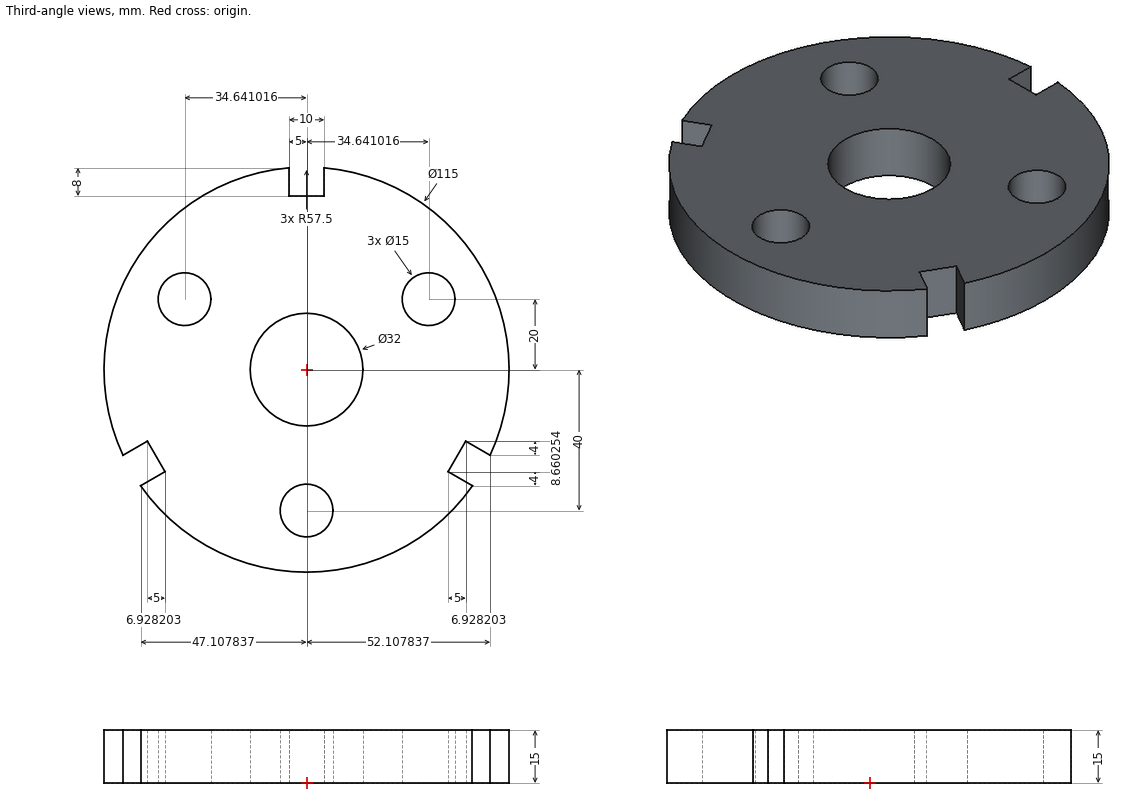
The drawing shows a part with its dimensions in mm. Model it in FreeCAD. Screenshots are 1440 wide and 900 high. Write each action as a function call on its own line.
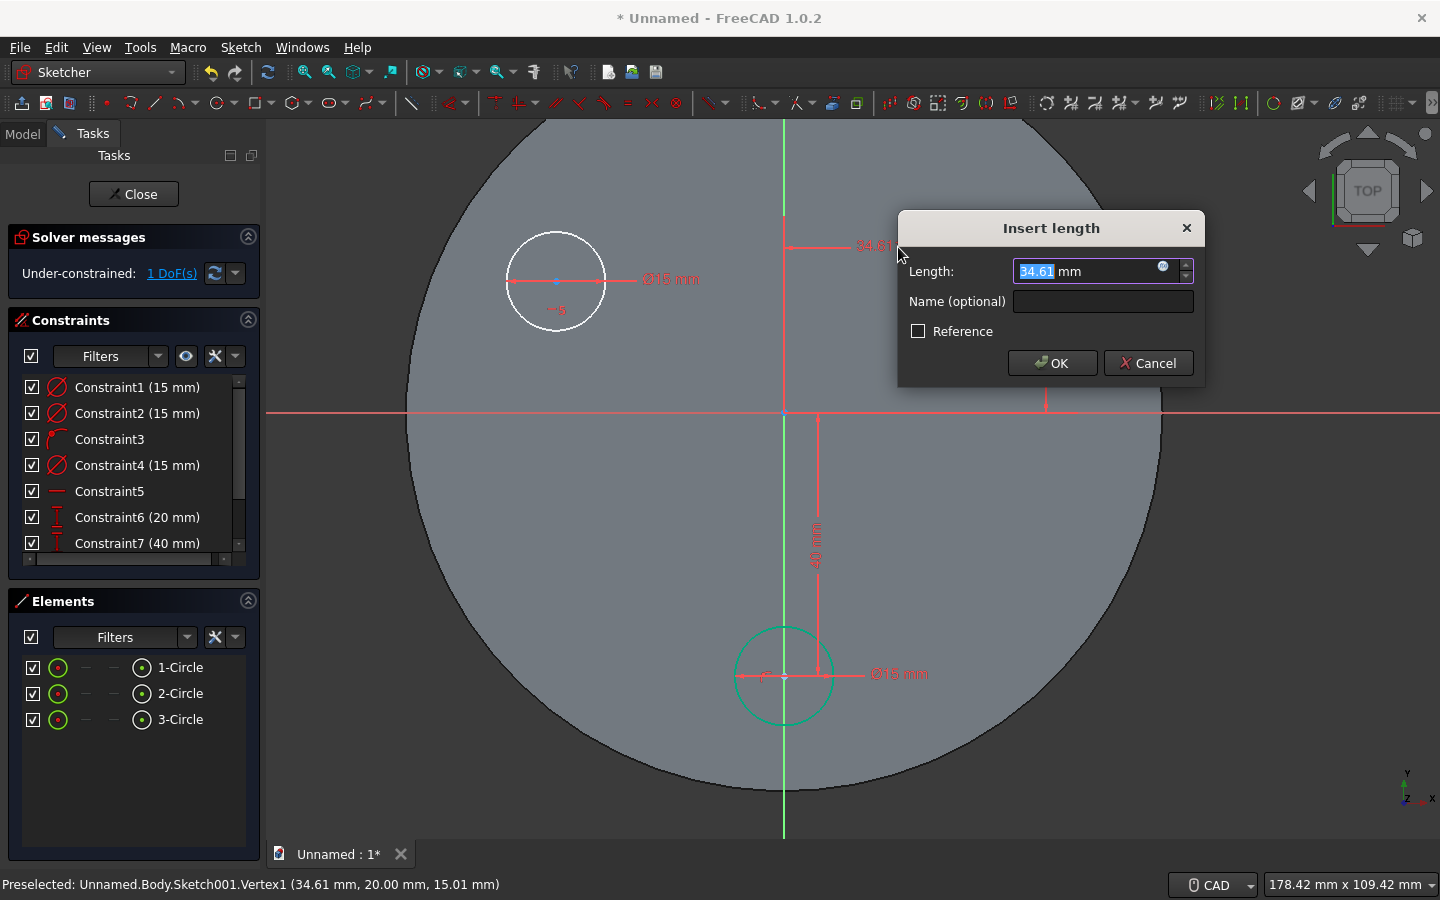
text(34.641016)
key(Return)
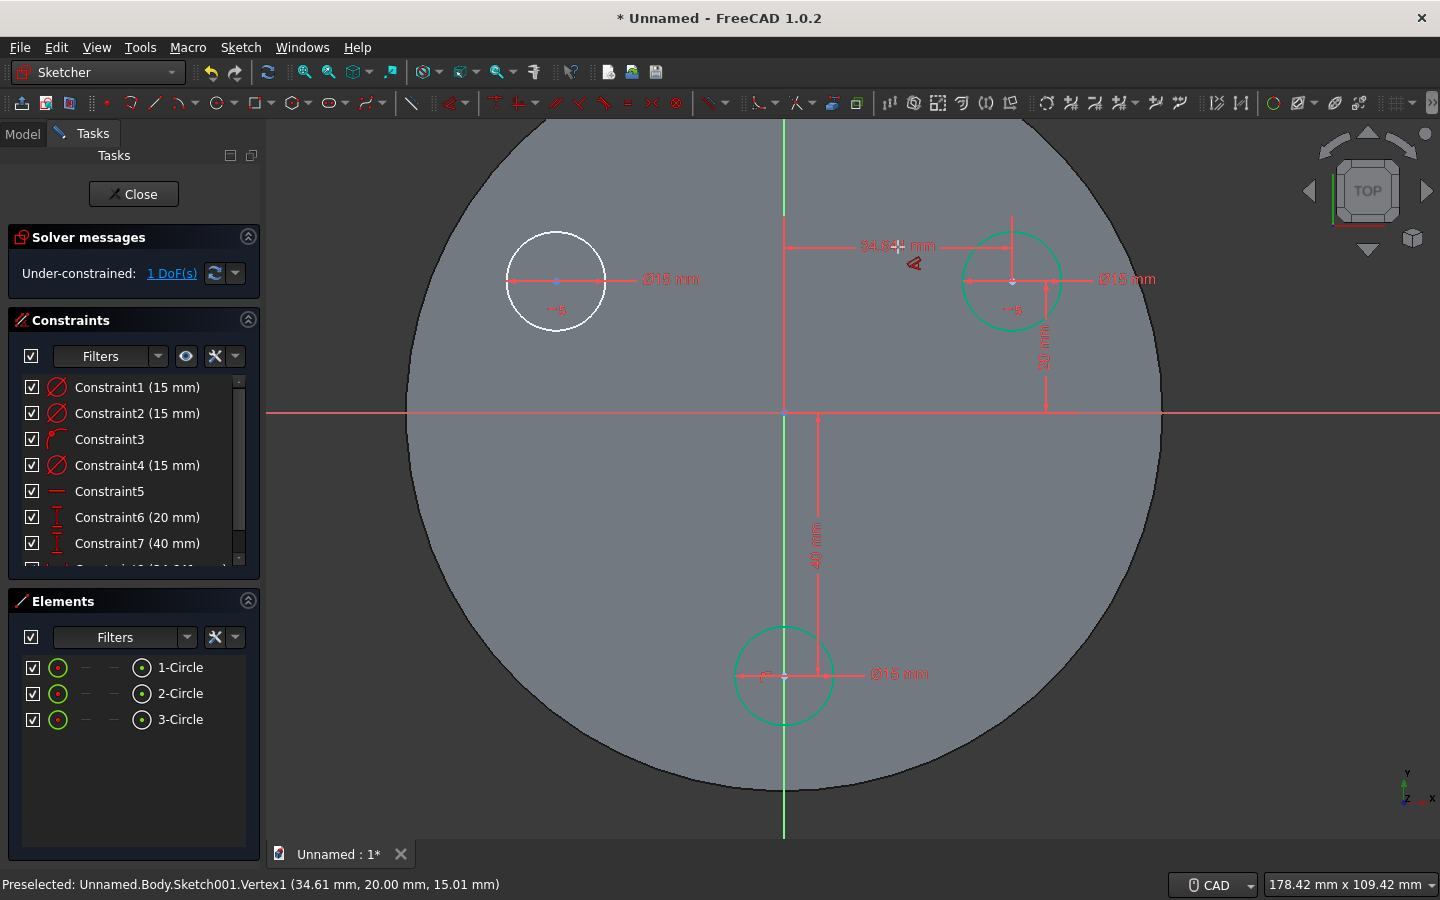
click(556, 281)
click(670, 247)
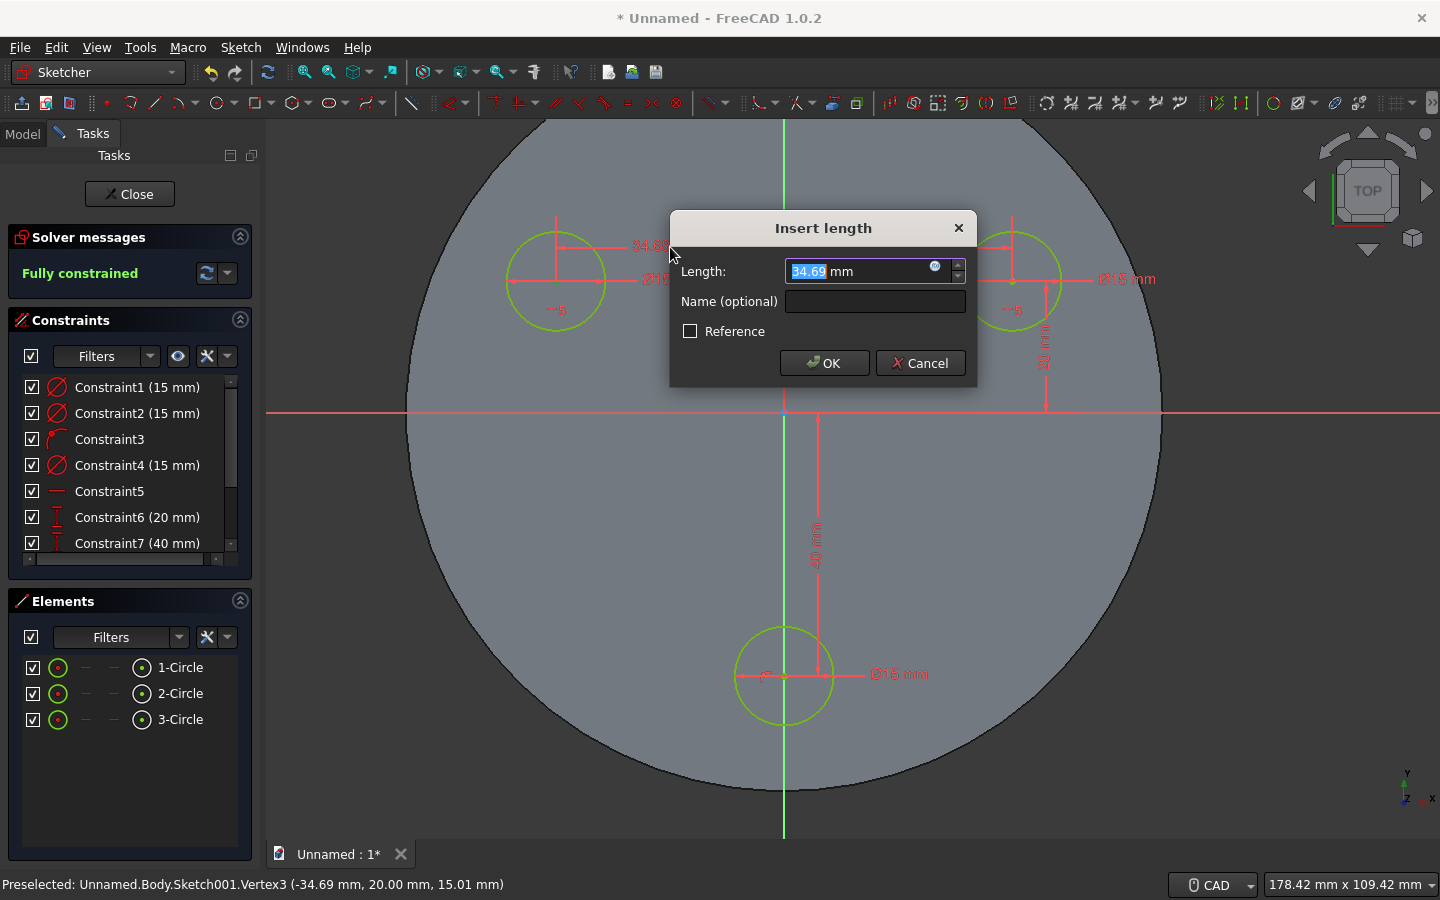
text(34.641016)
key(Return)
key(Escape)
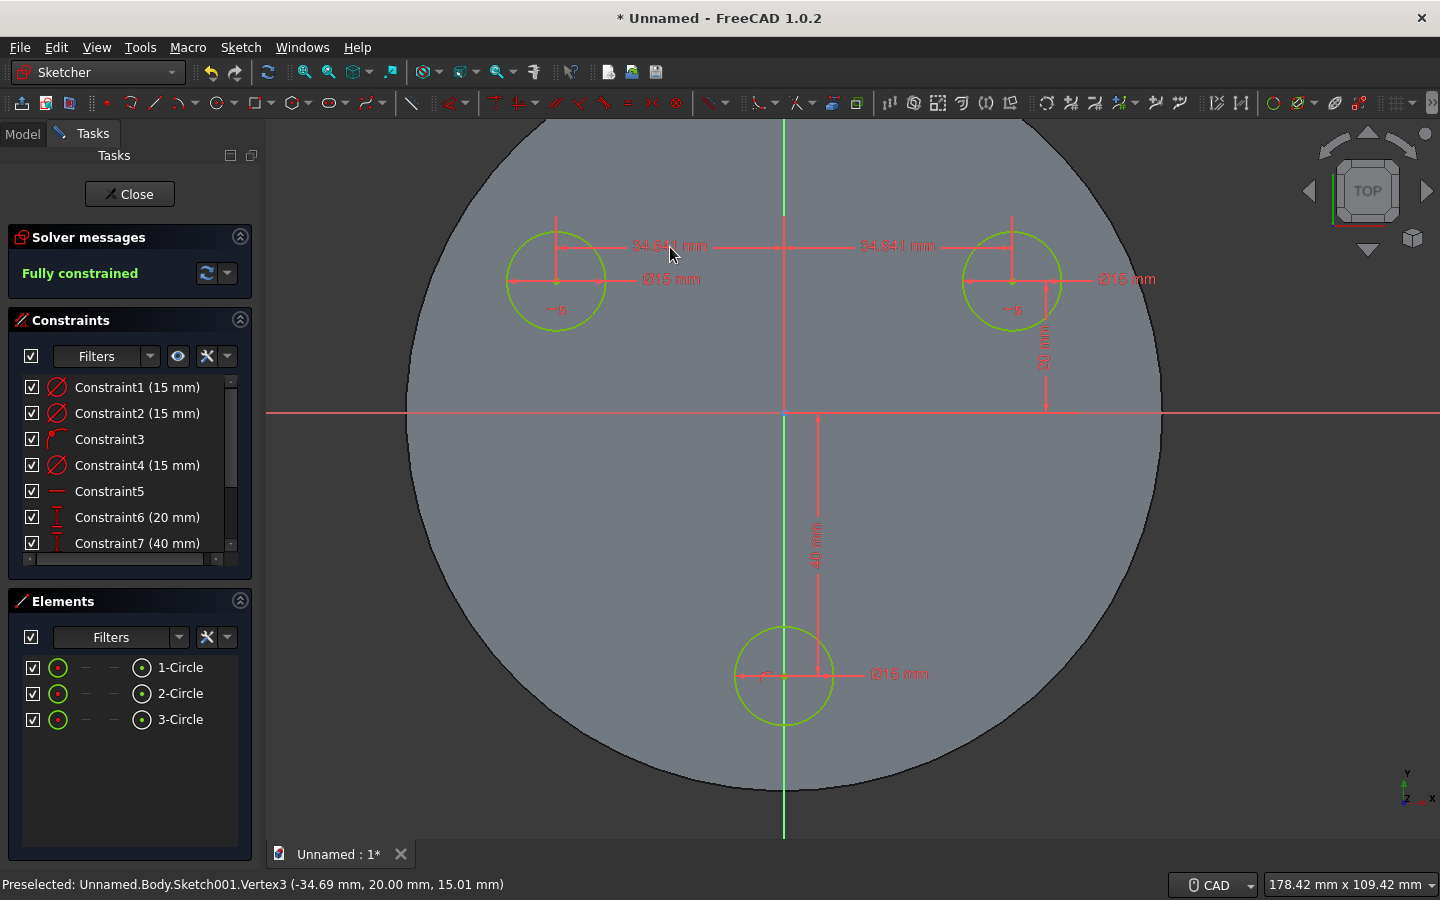
click(130, 194)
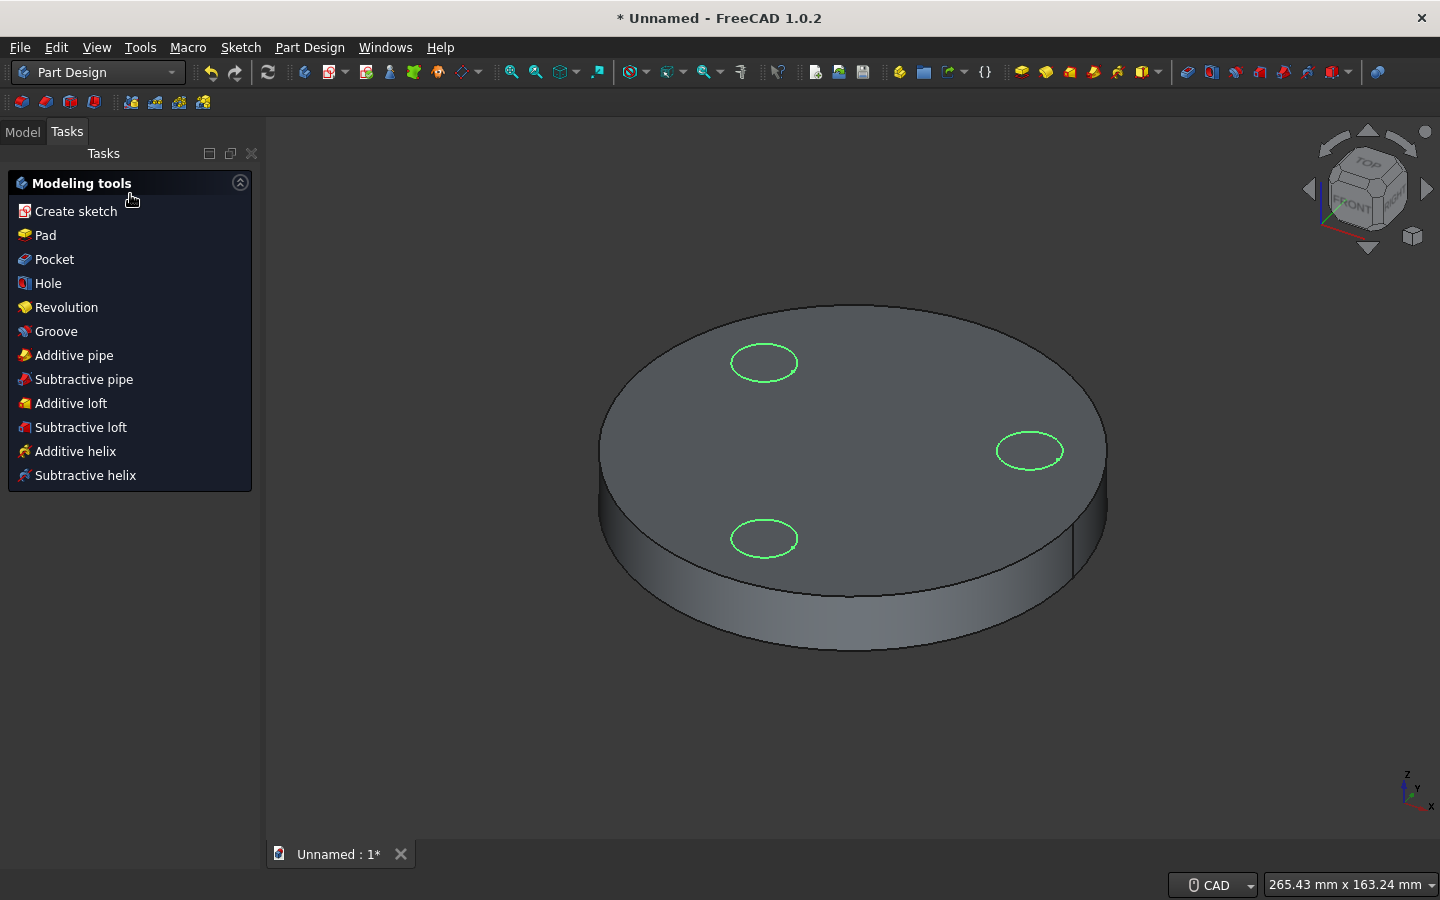
click(1188, 72)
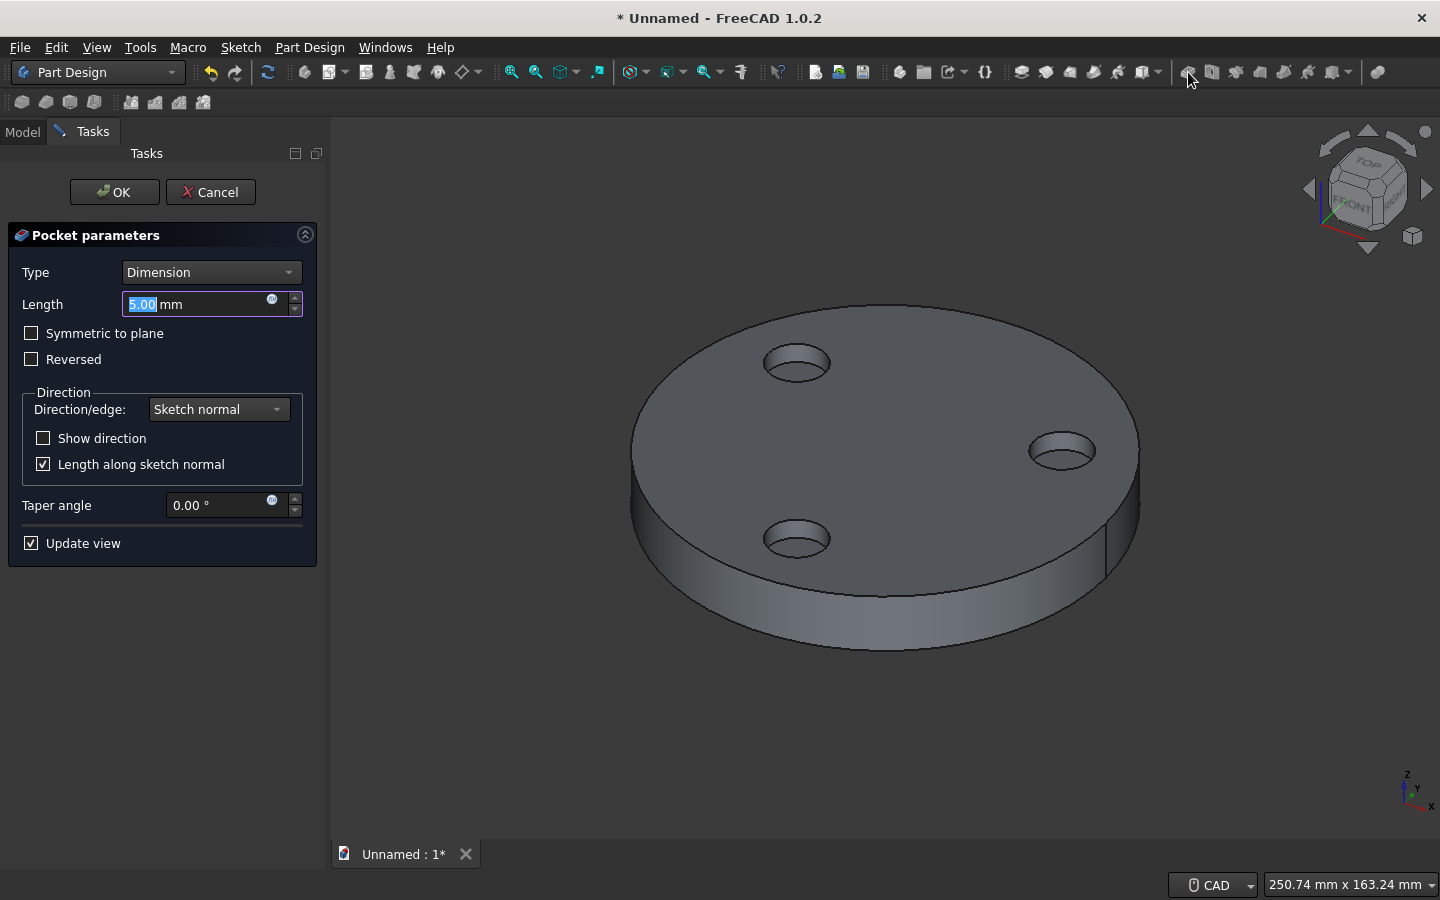
text(15)
key(Tab)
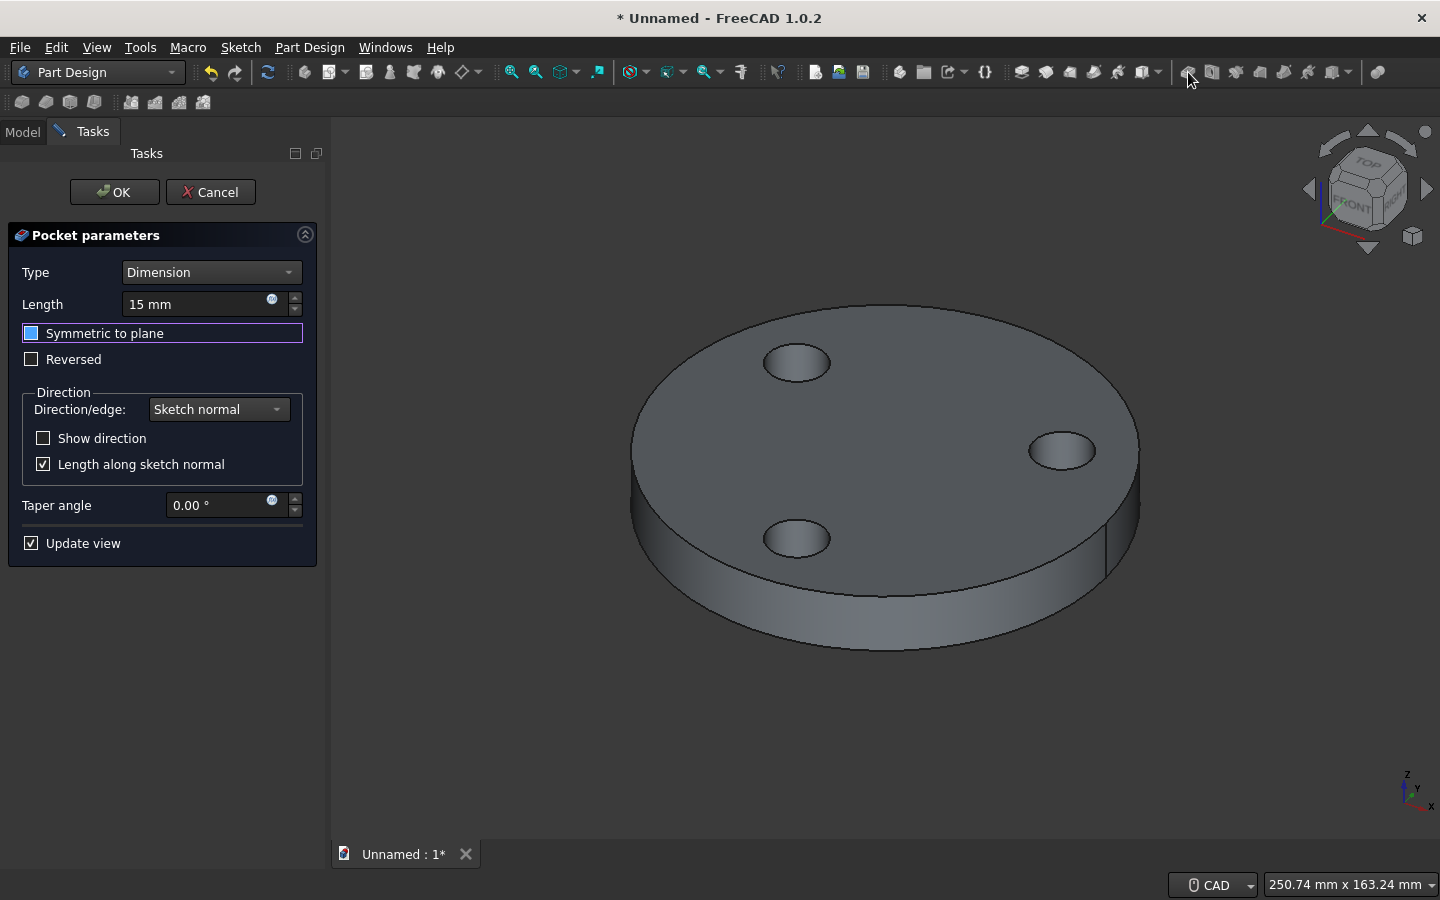
click(115, 192)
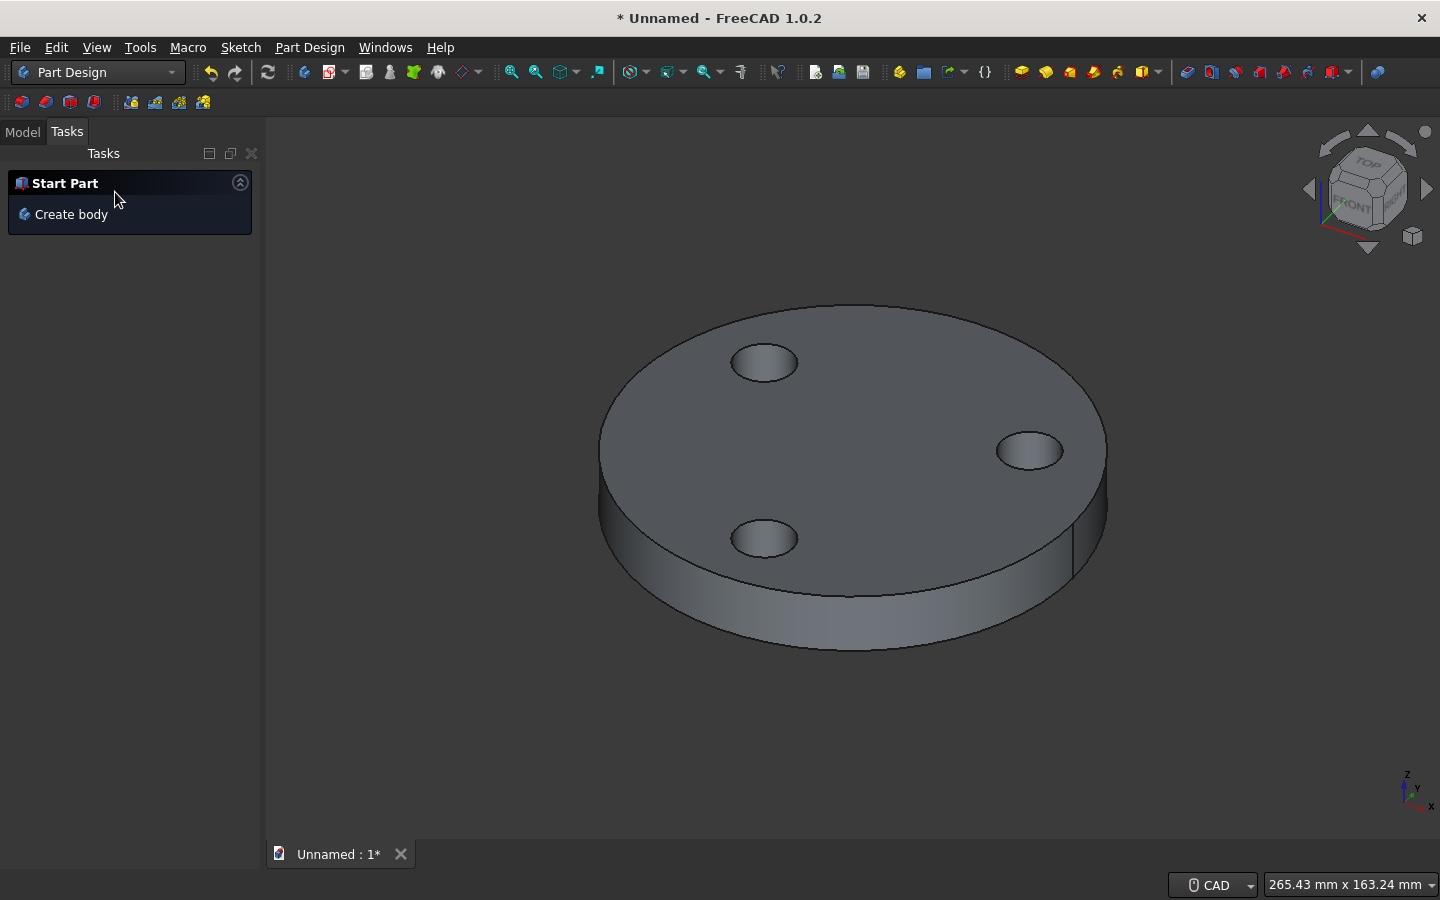
click(853, 450)